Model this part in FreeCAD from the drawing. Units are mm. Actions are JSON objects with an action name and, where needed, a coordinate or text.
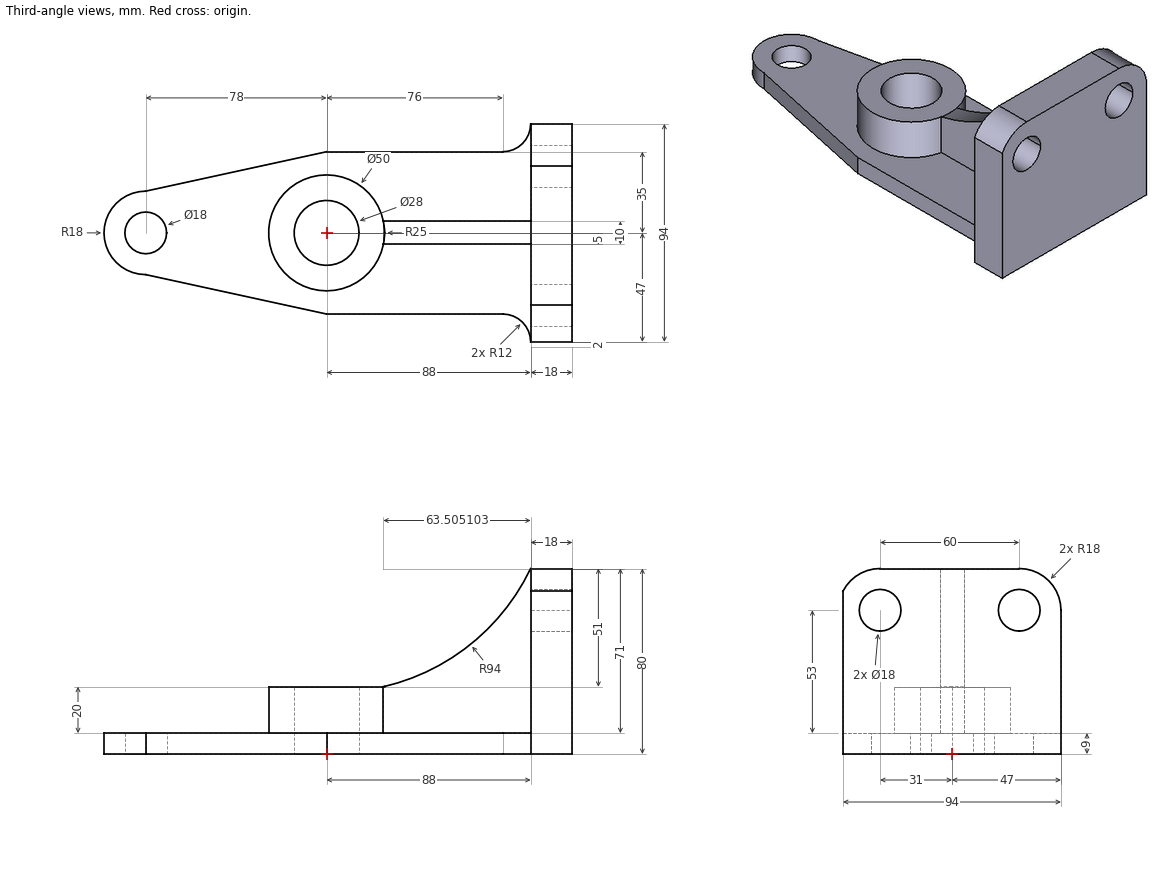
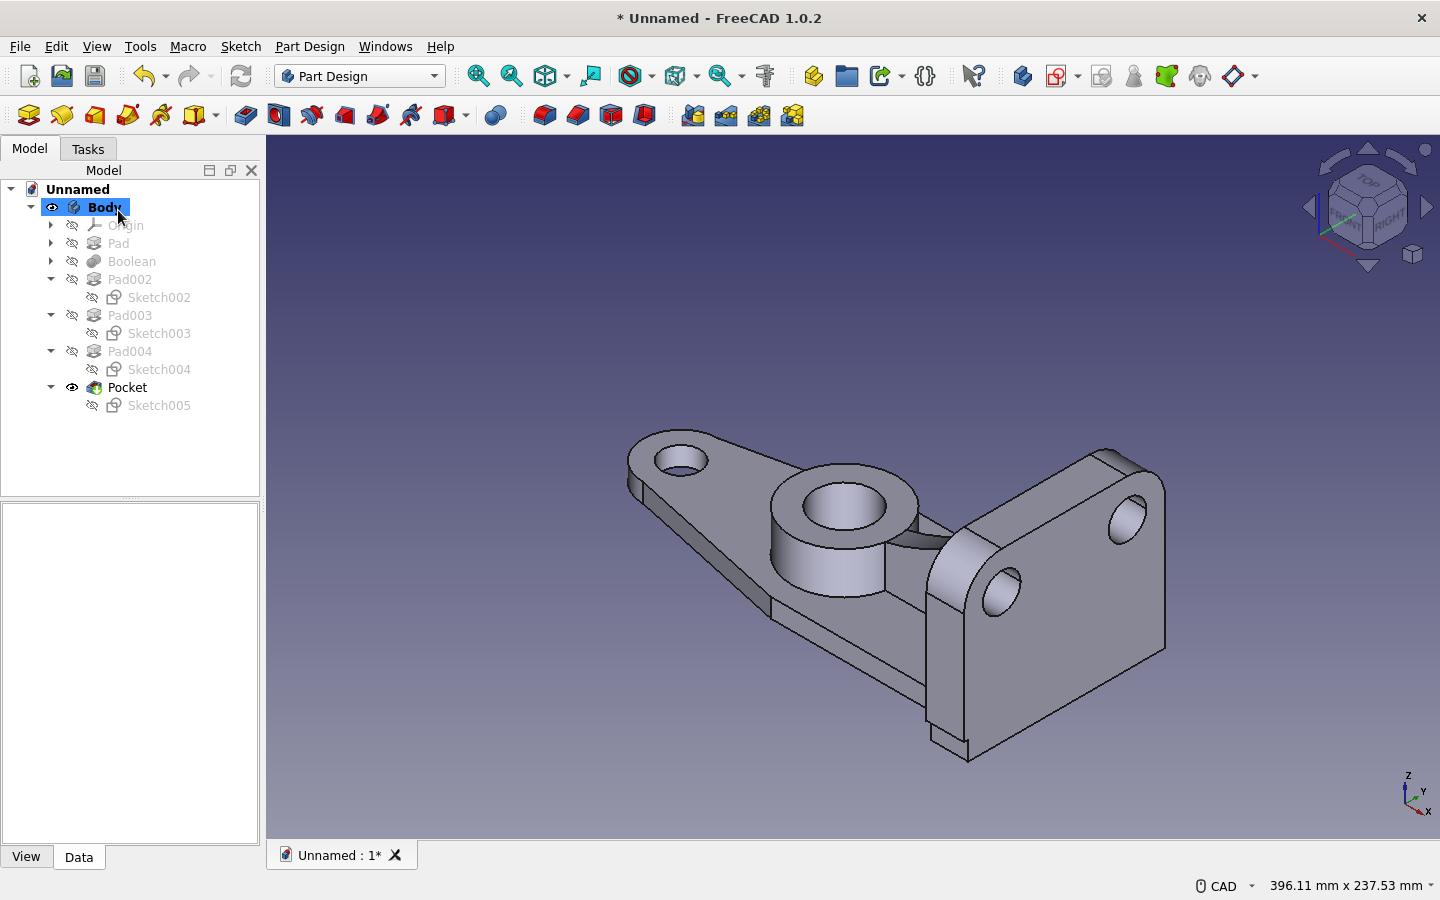
{"action": "left_click", "coordinate": [726, 485]}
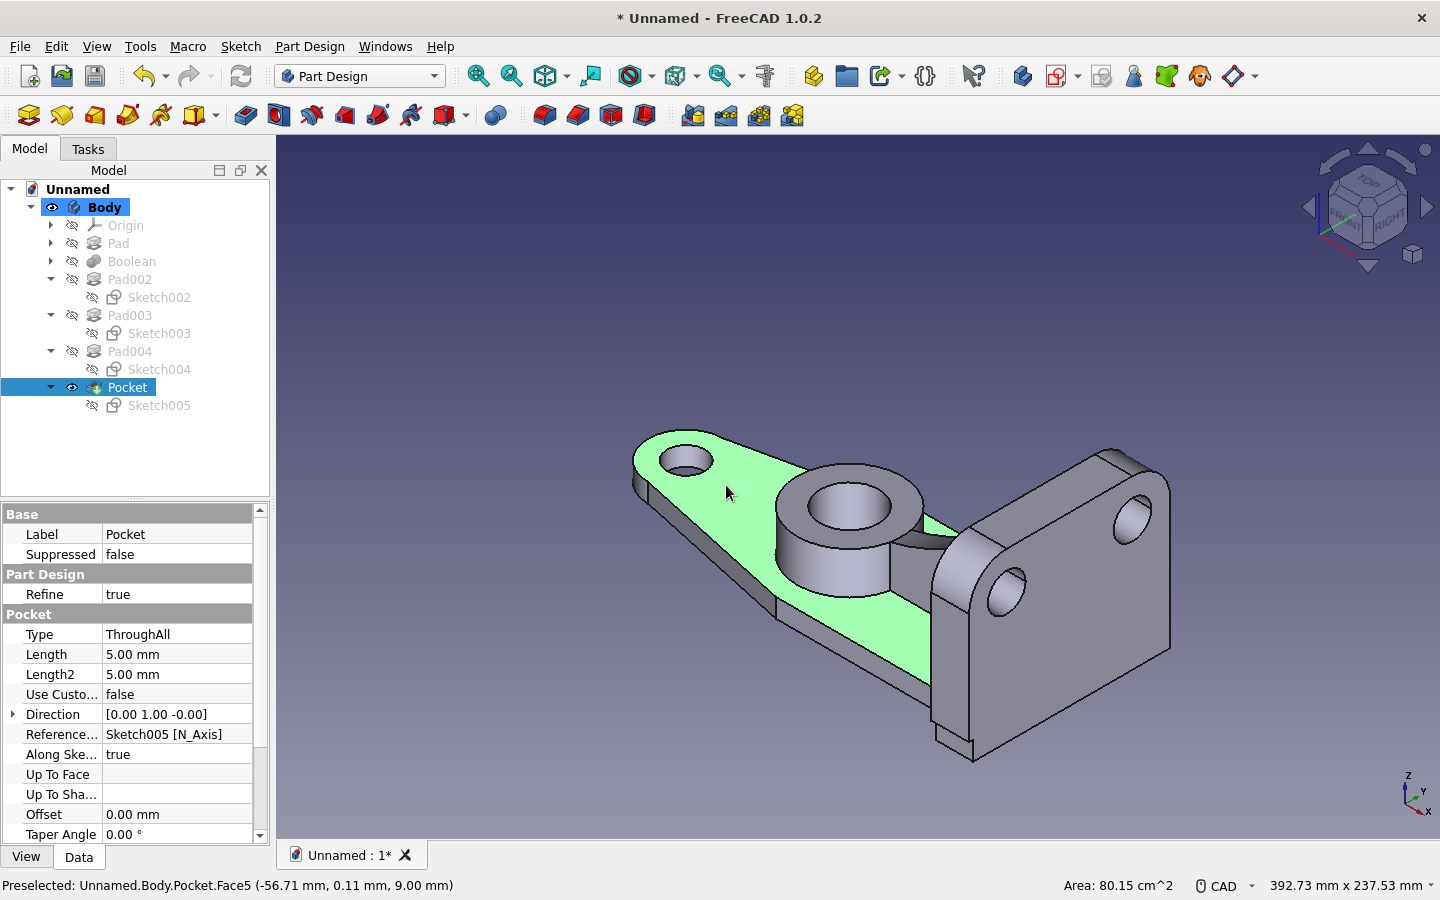
{"action": "left_click", "coordinate": [1056, 76]}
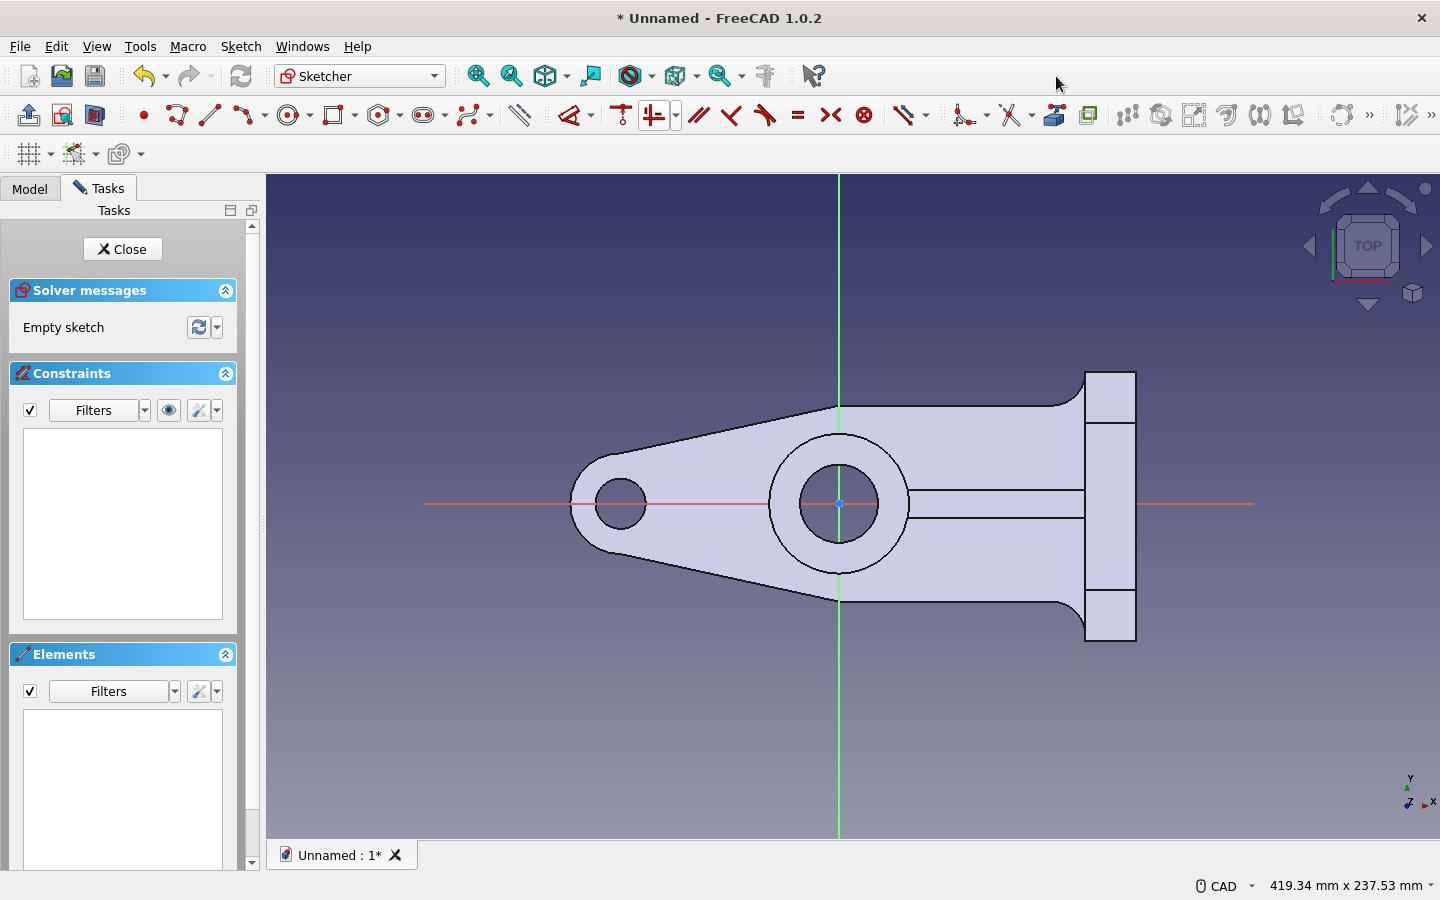
{"action": "left_click", "coordinate": [95, 116]}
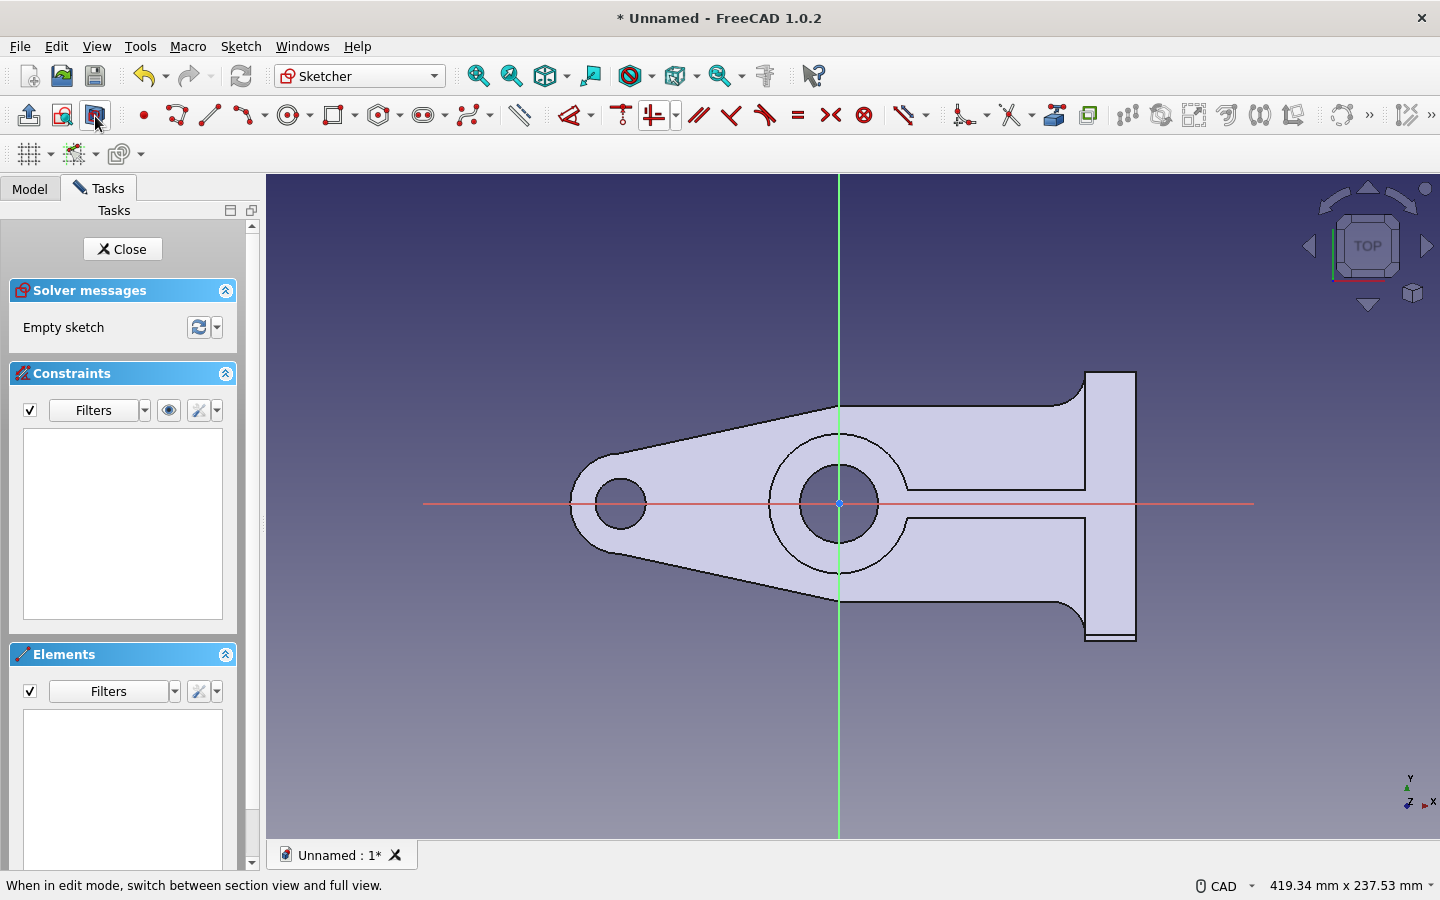
{"action": "scroll", "coordinate": [1137, 649], "scroll_direction": "up", "scroll_amount": 13}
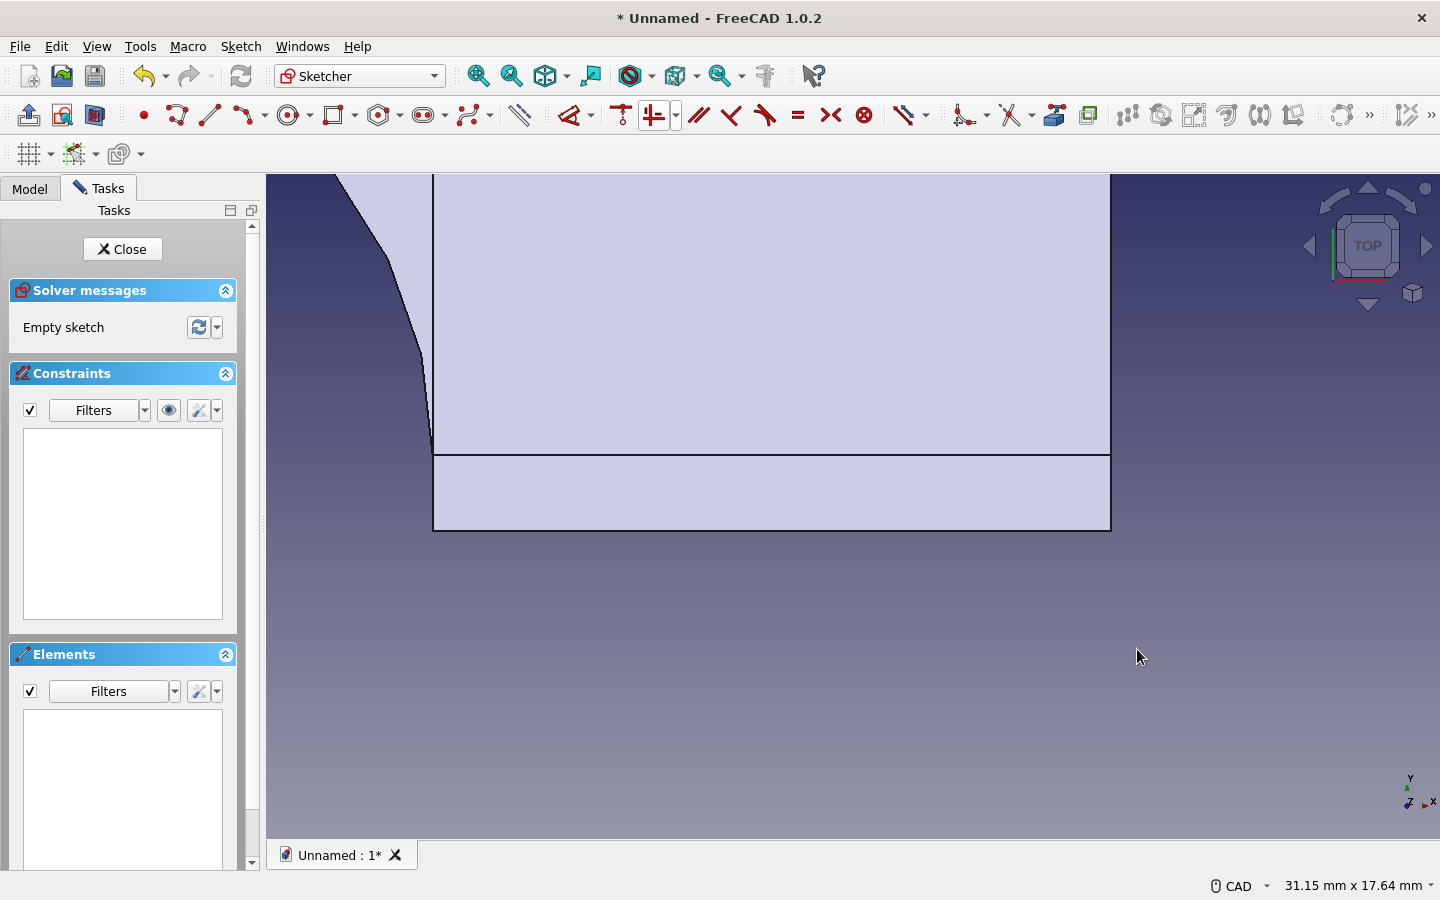
{"action": "left_click", "coordinate": [332, 116]}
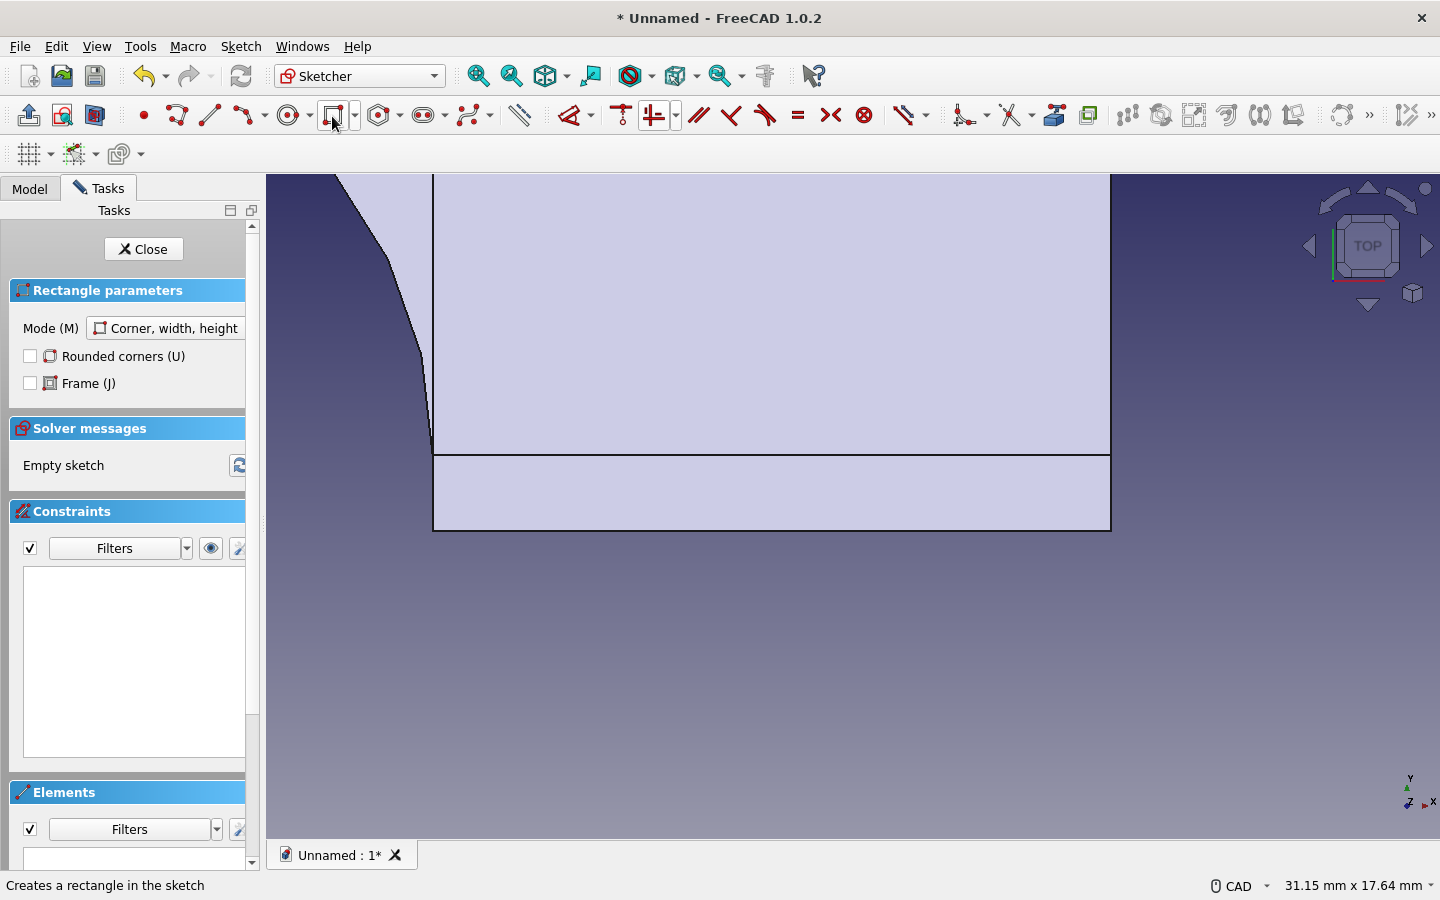
{"action": "left_click", "coordinate": [433, 455]}
{"action": "left_click", "coordinate": [1111, 531]}
{"action": "key", "text": "Escape"}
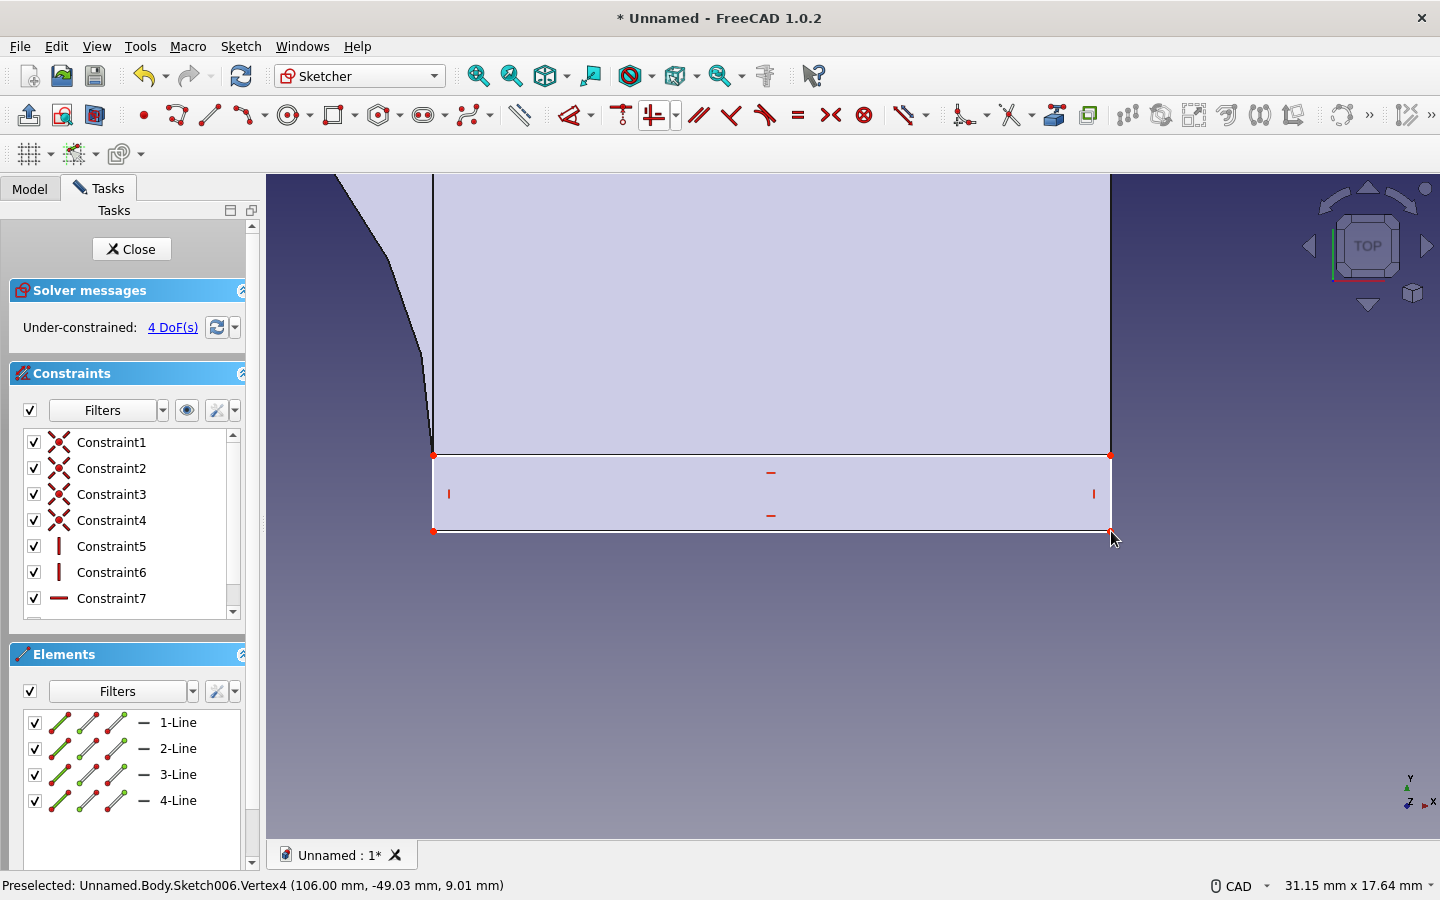
{"action": "left_click", "coordinate": [568, 116]}